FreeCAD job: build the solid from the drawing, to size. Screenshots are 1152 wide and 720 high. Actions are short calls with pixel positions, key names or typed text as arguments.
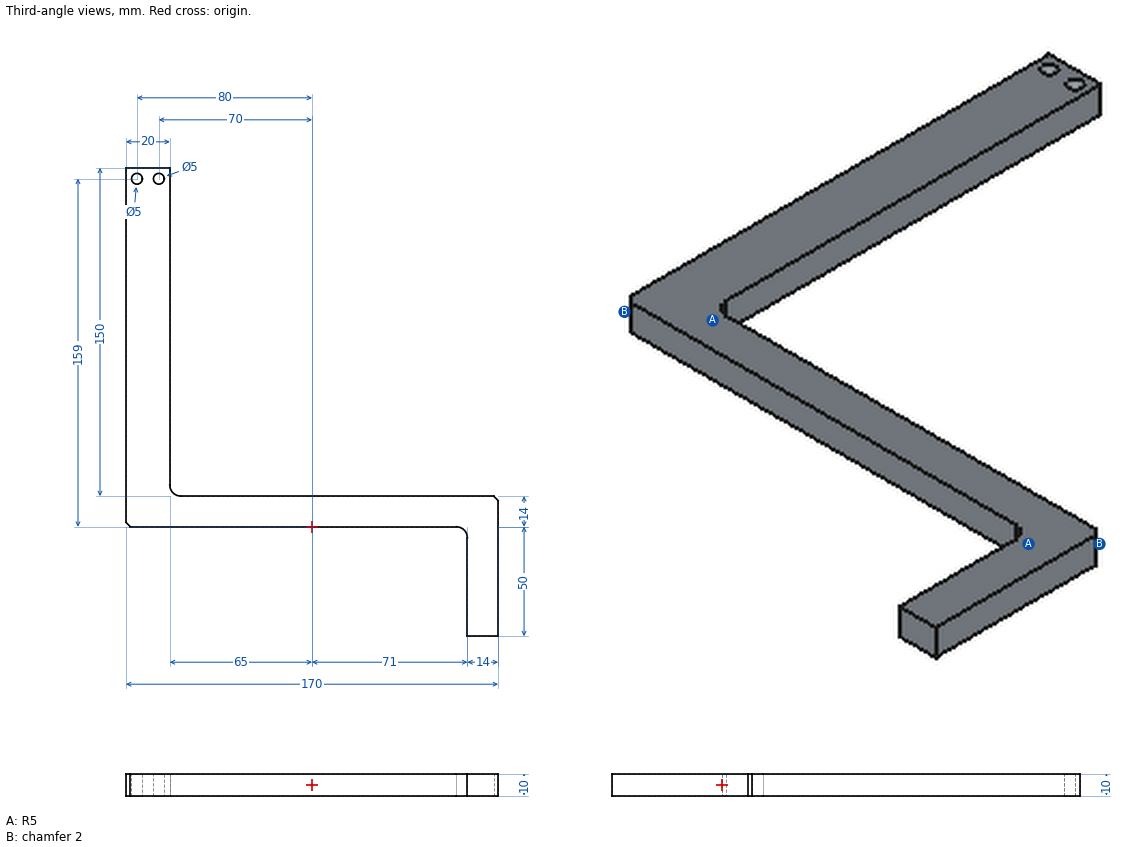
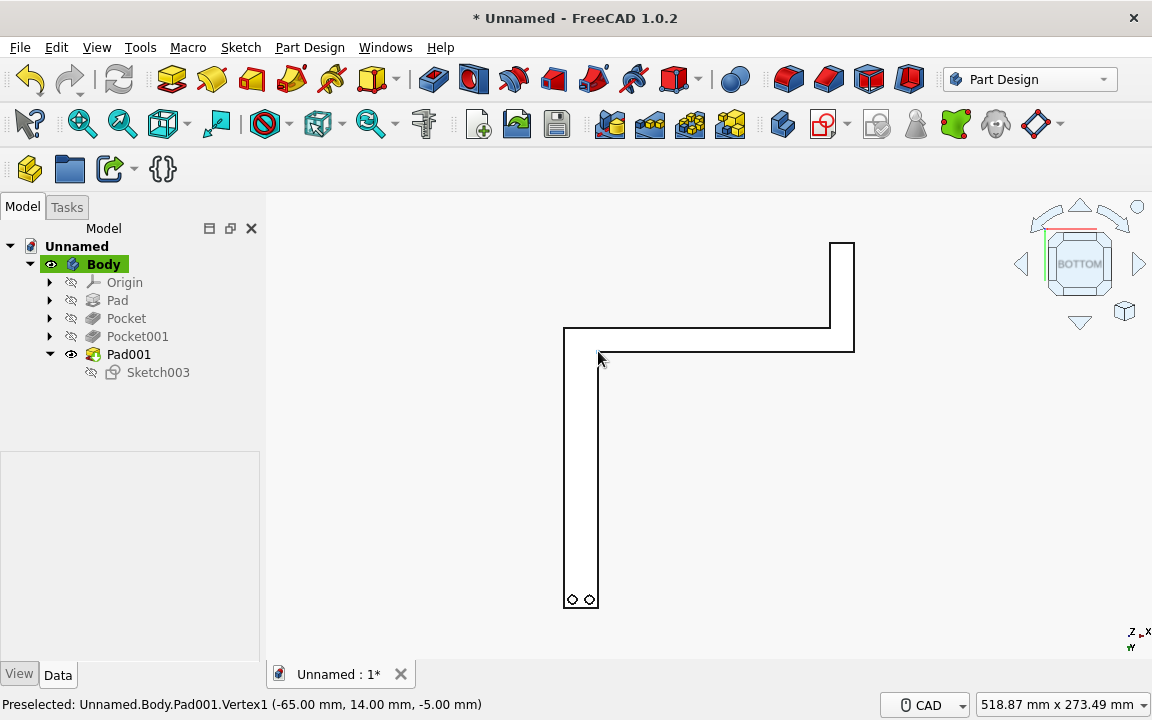
key(4)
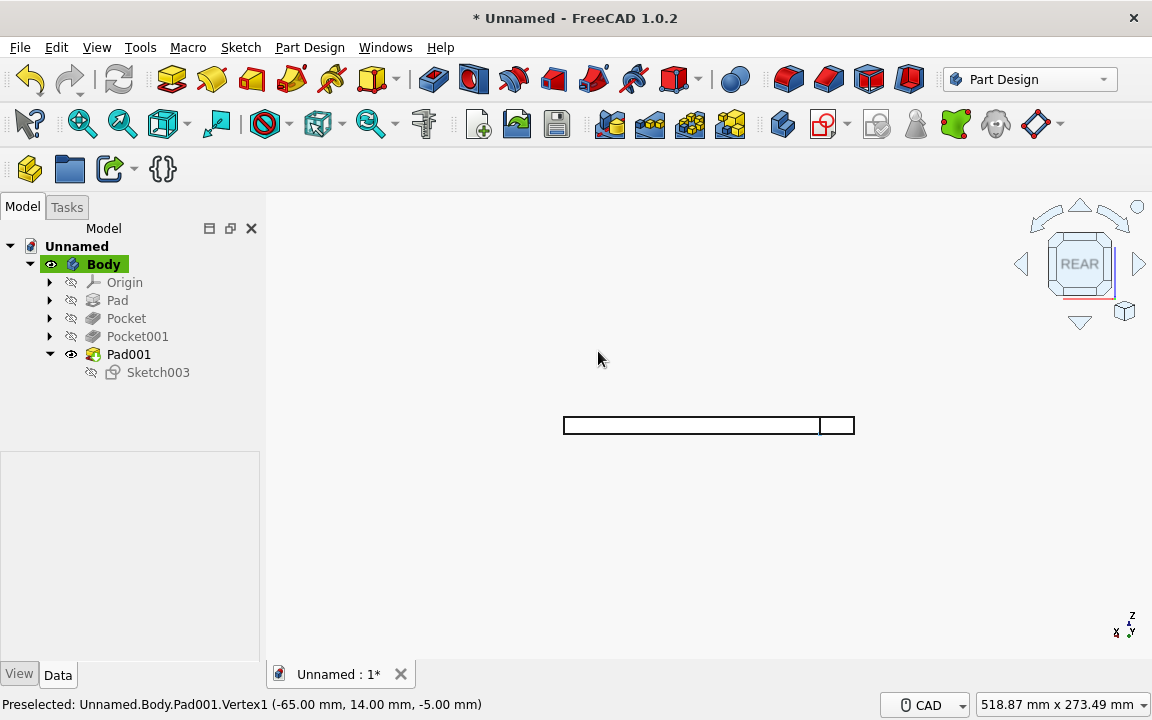
key(v)
key(f)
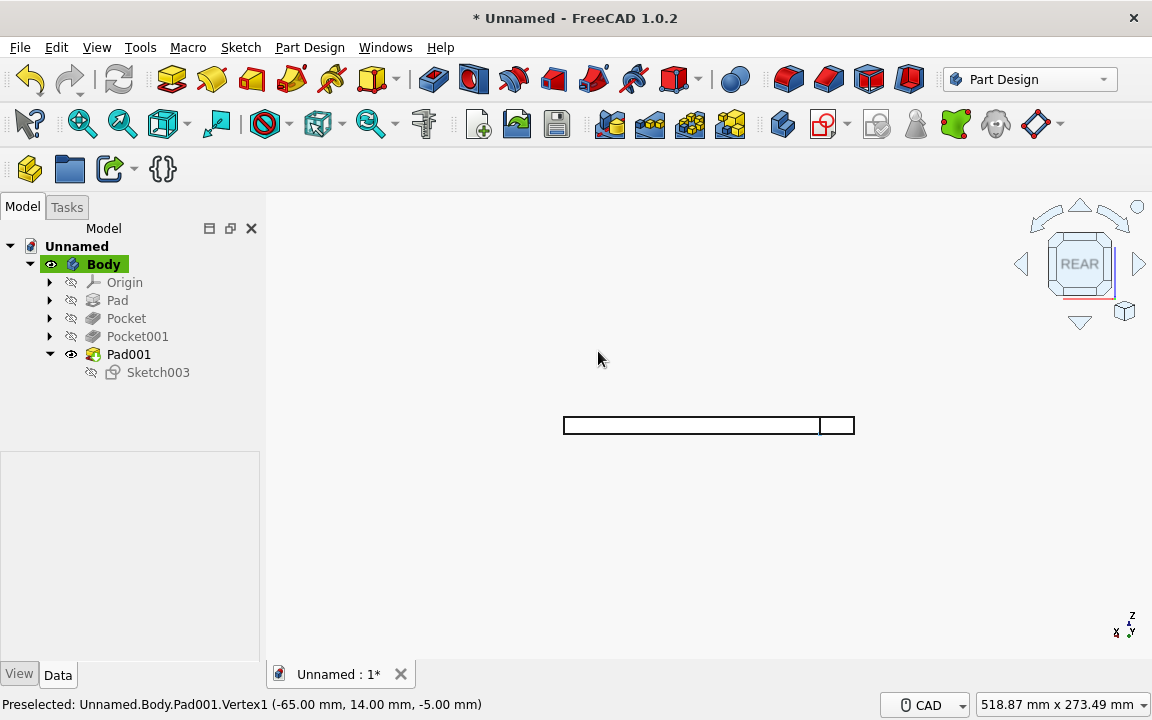
scroll(820, 425, up, 5)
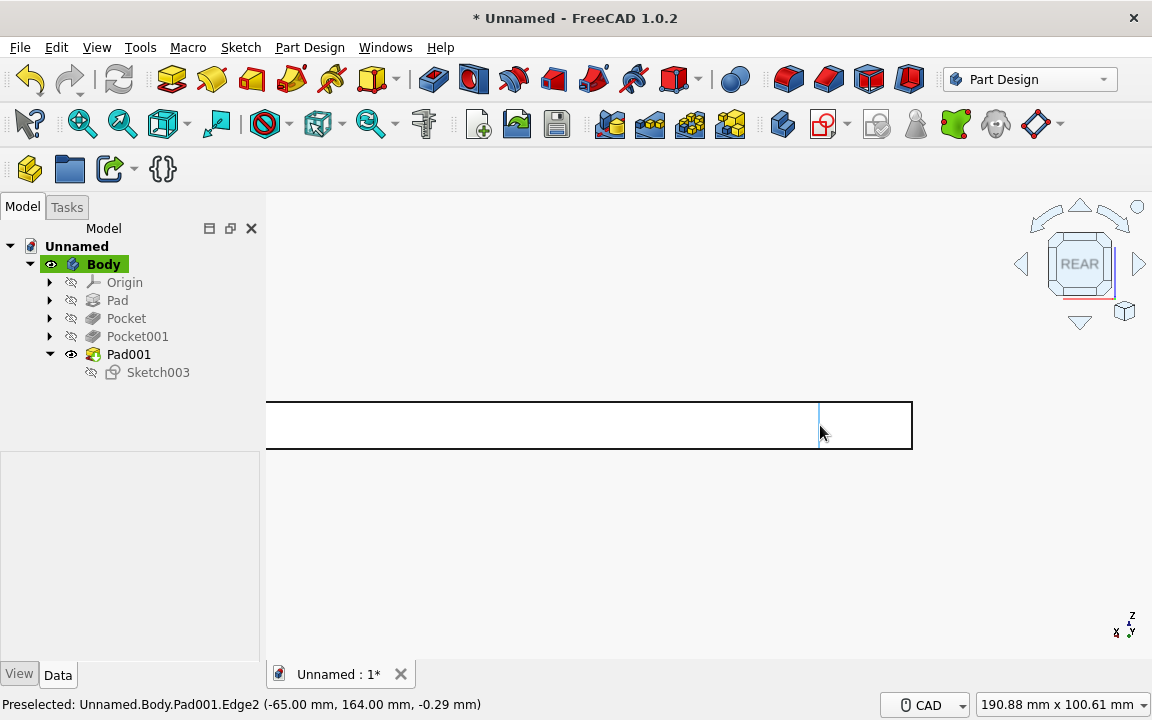
key(v)
key(f)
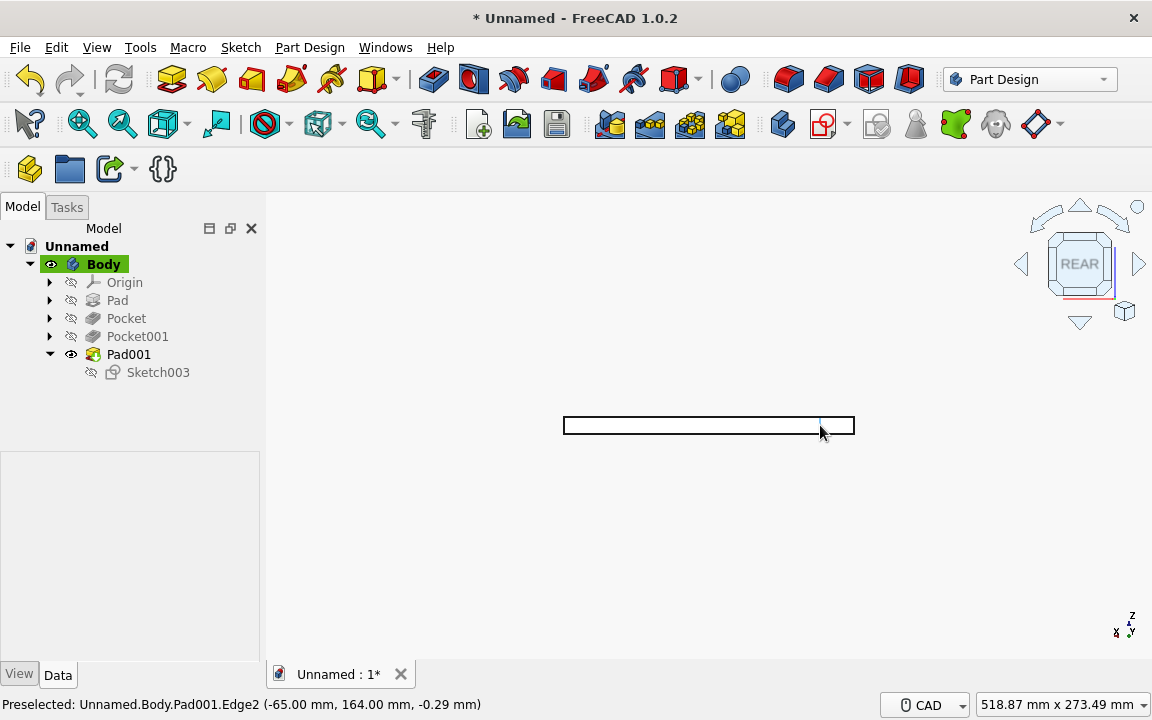
key(6)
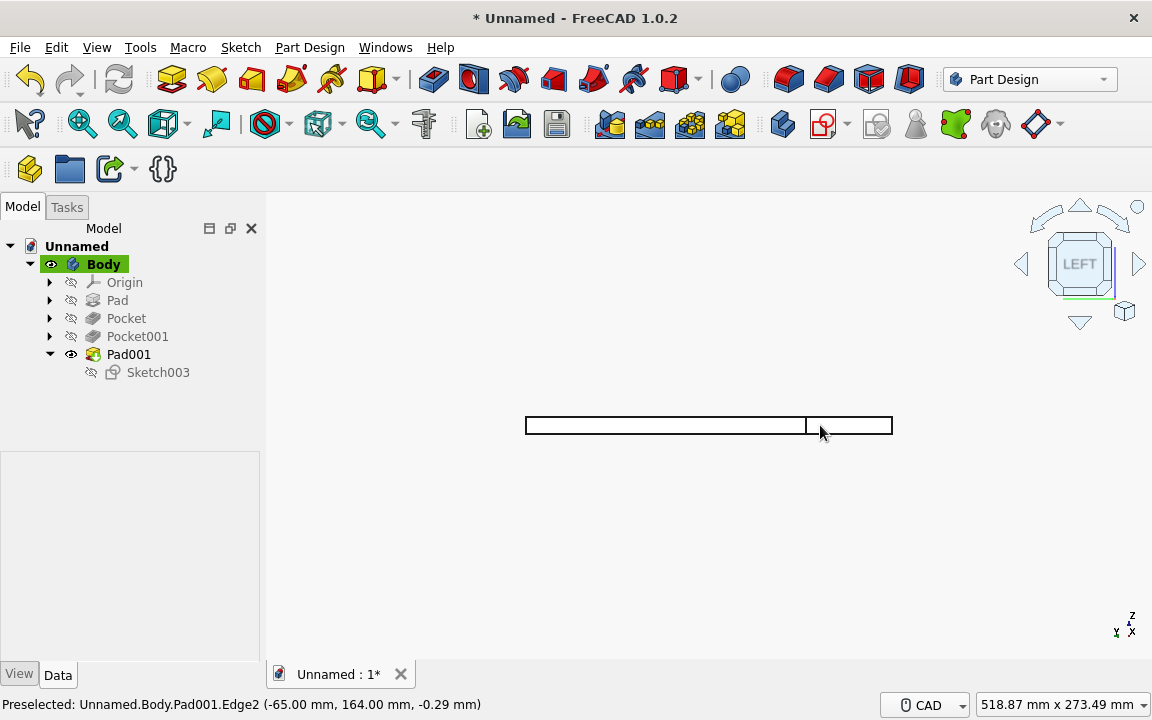
click(84, 124)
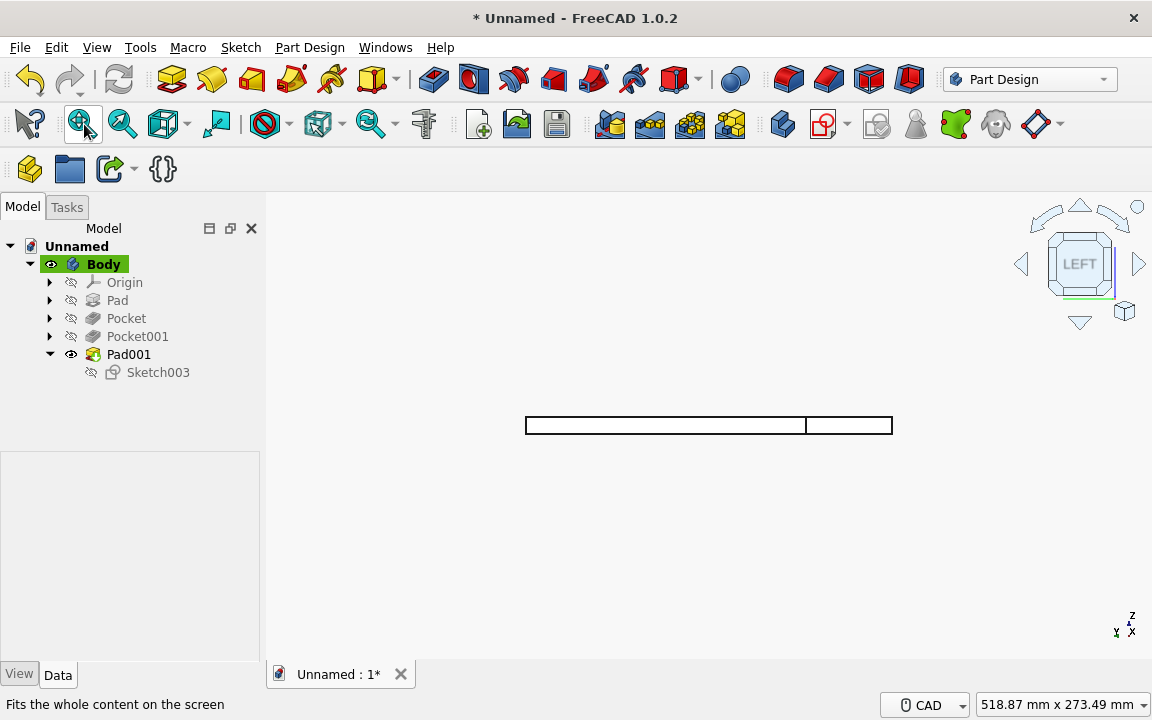
scroll(782, 424, up, 5)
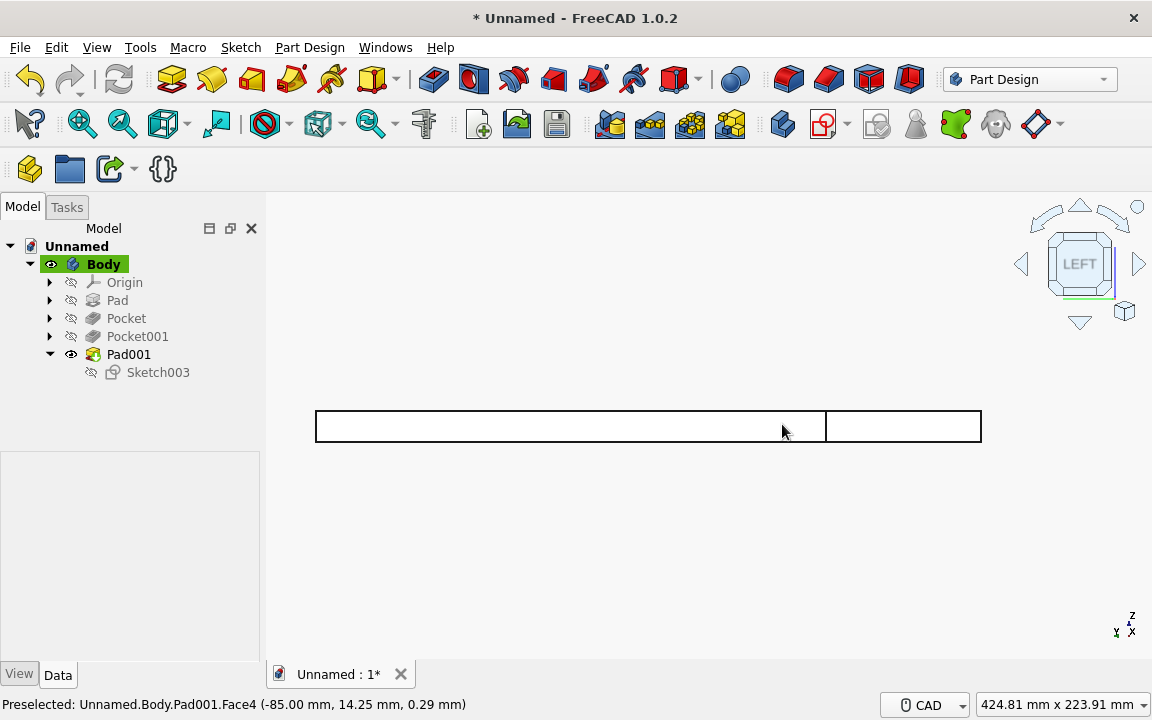
click(84, 124)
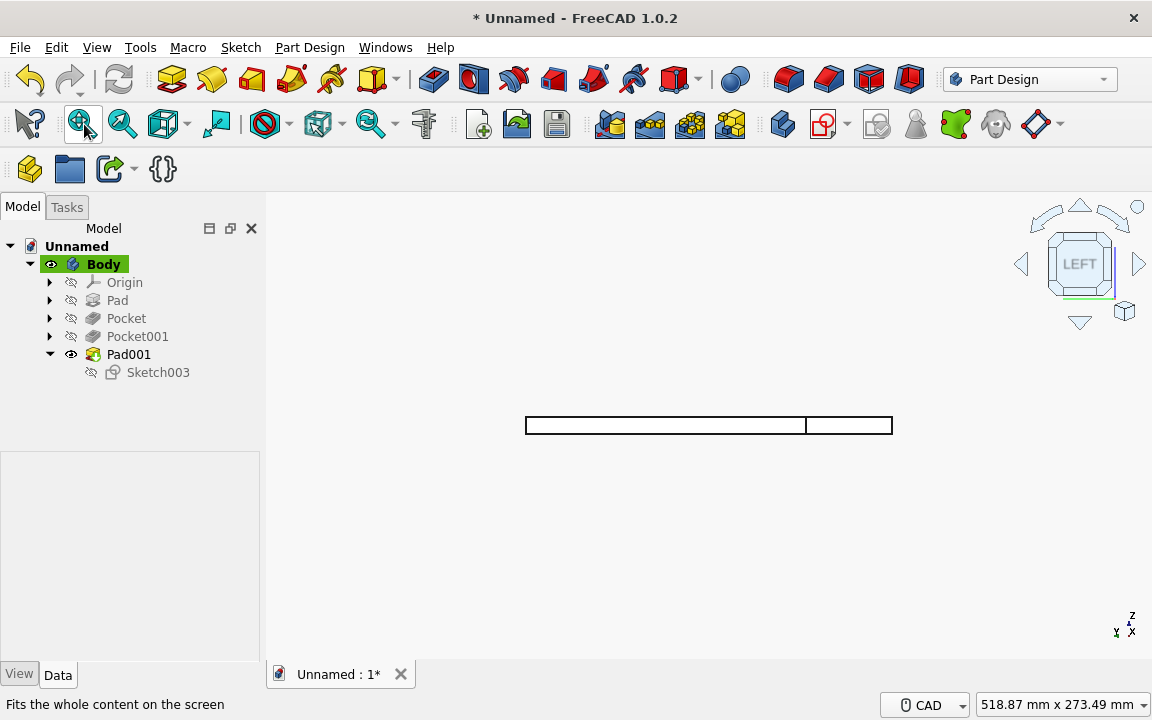
key(v)
key(3)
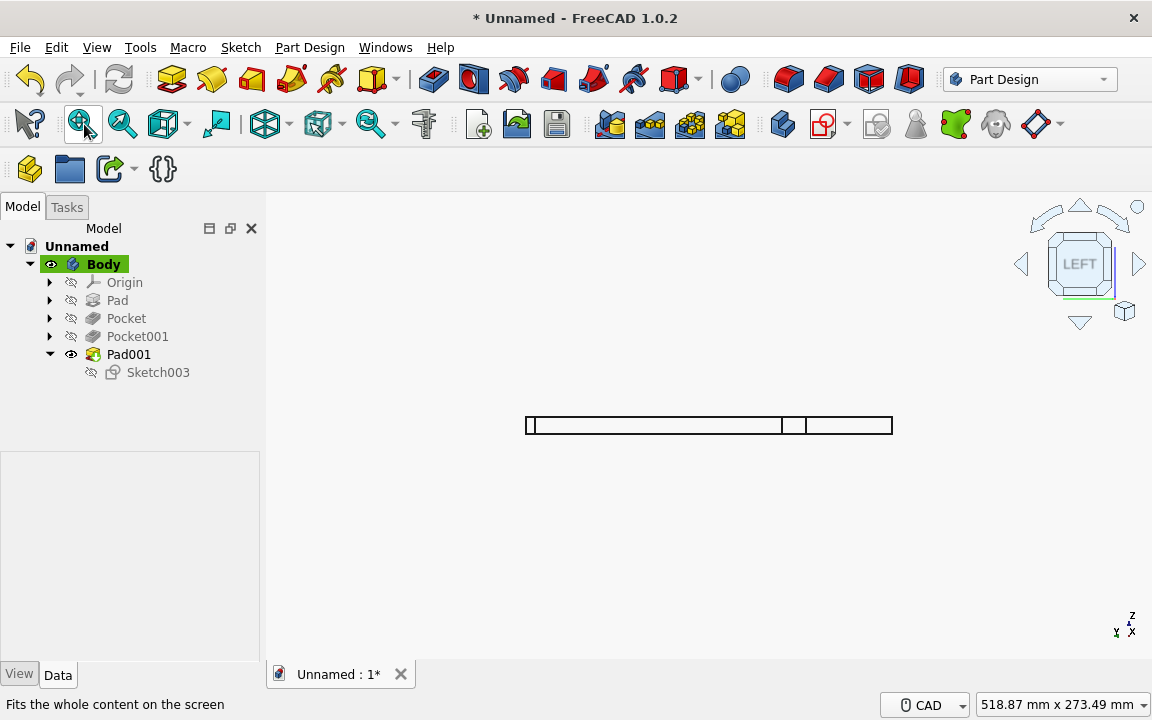
key(0)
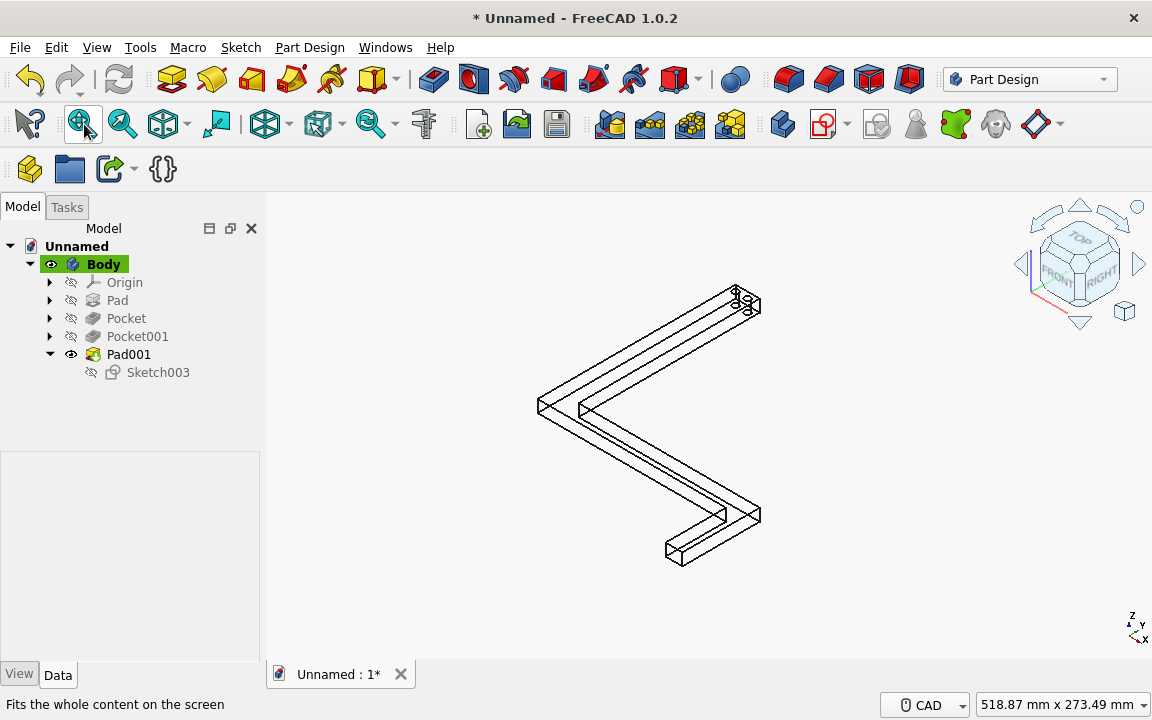
click(579, 411)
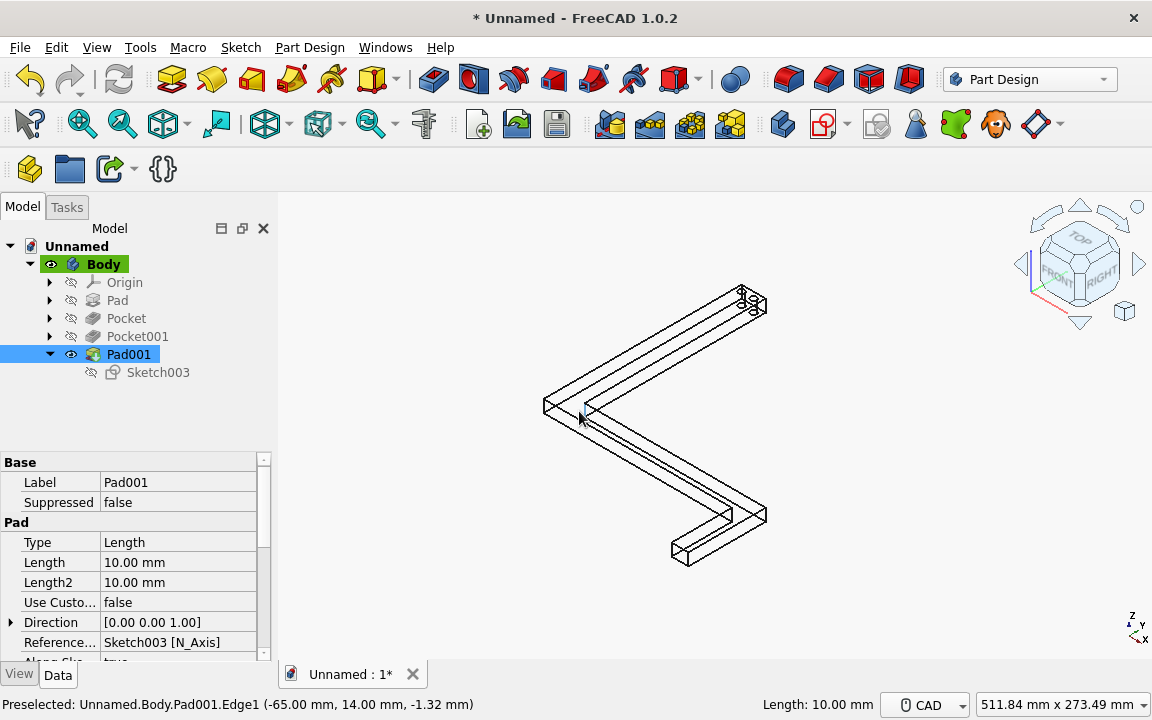
click(732, 515, ctrl)